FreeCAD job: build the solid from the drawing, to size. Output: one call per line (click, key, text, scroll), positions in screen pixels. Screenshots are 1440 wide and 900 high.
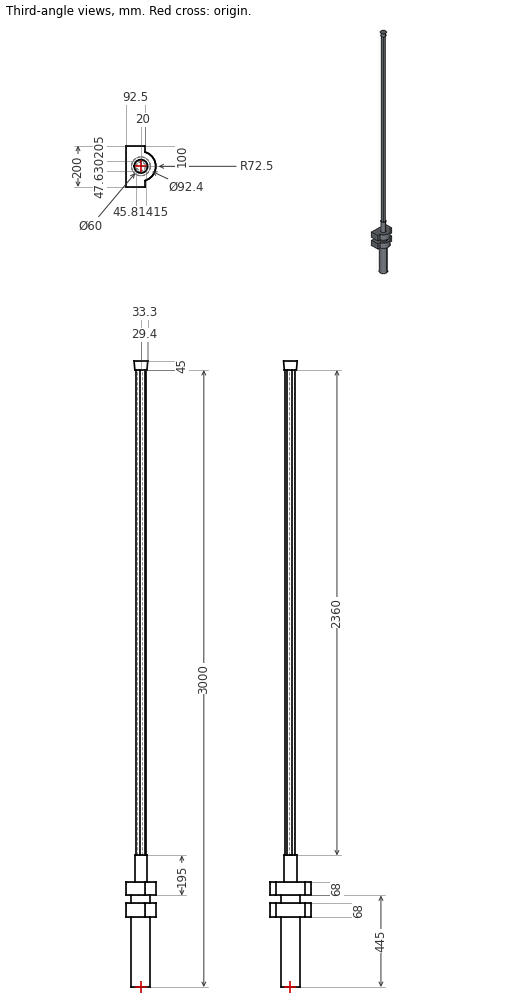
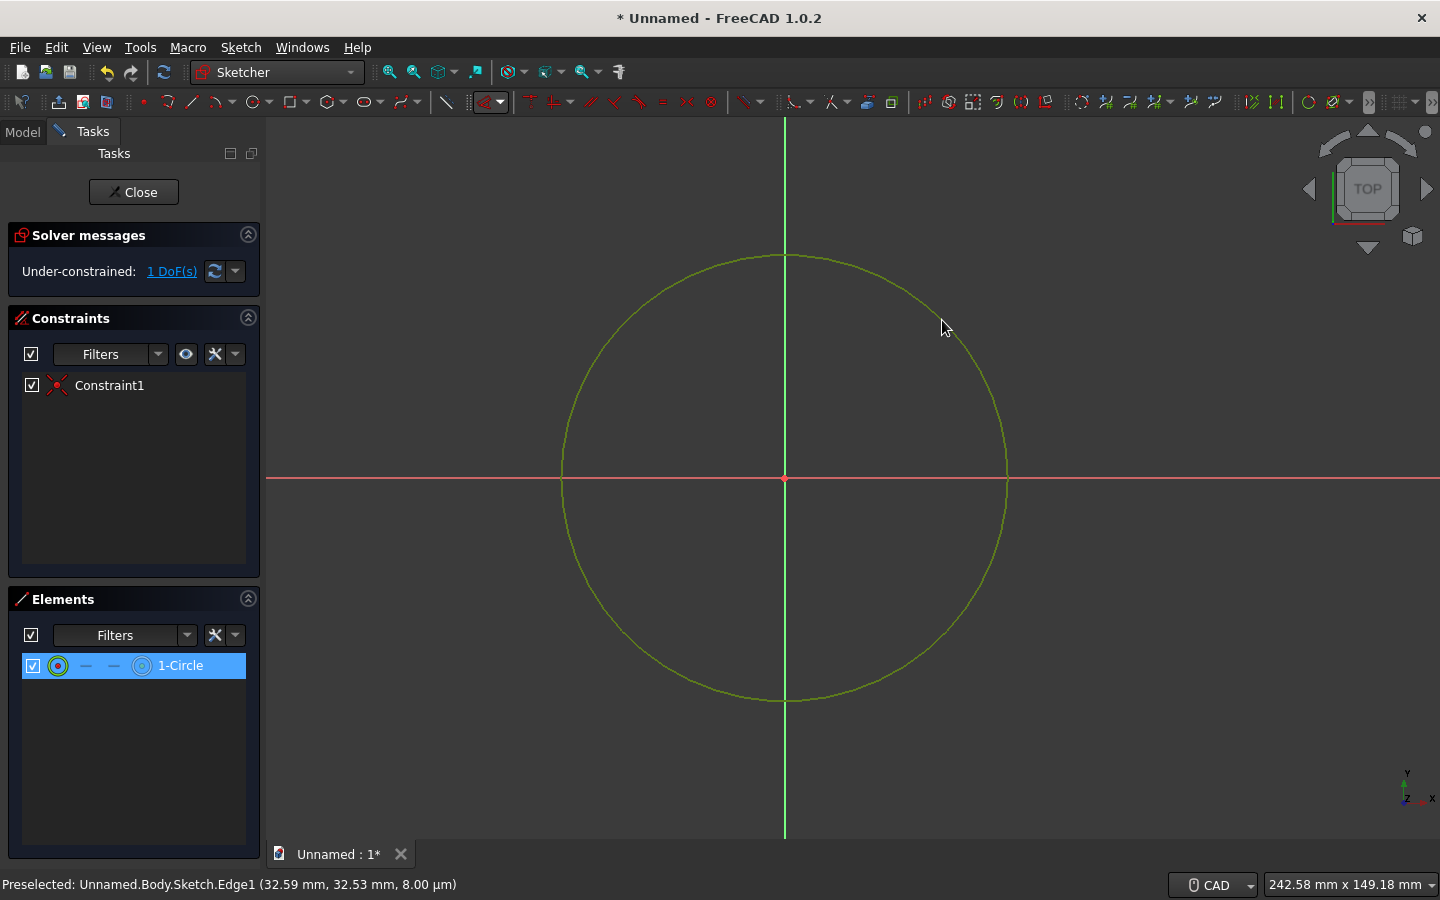
key(k)
key(o)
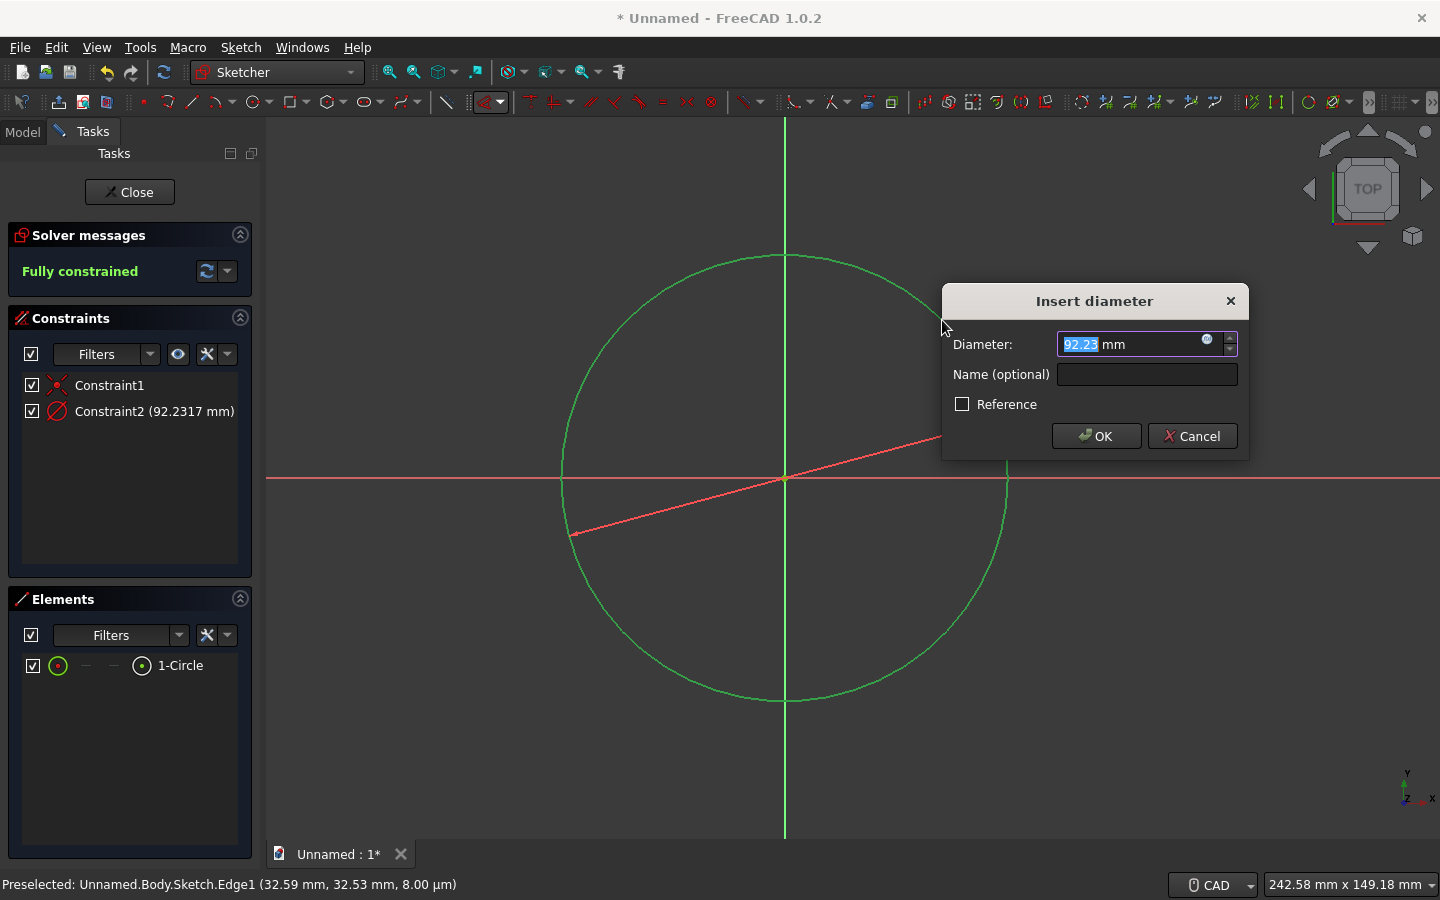
text(92.4)
key(Return)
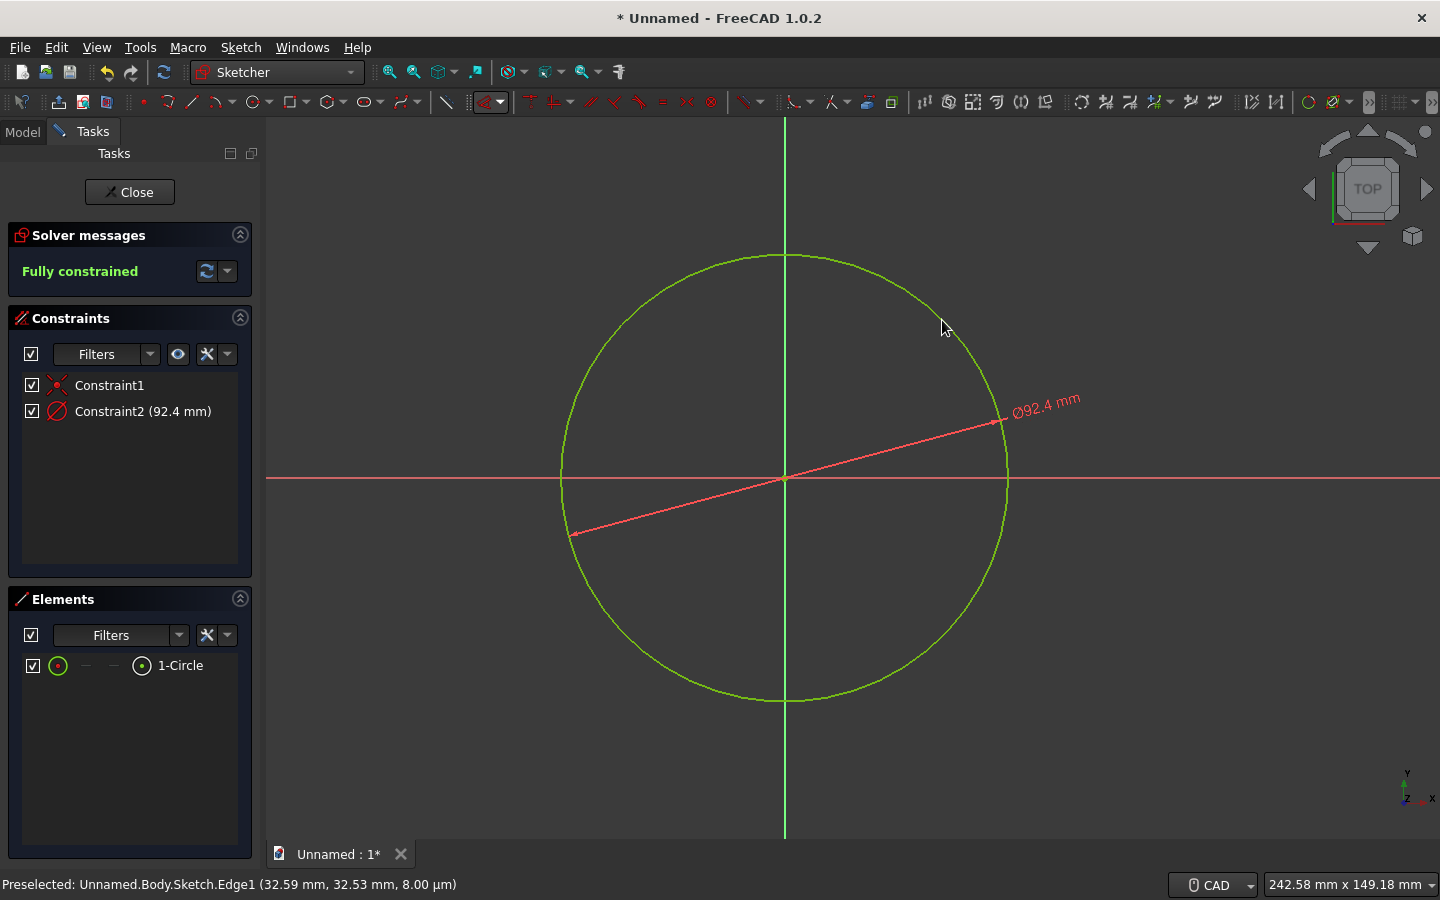
click(130, 192)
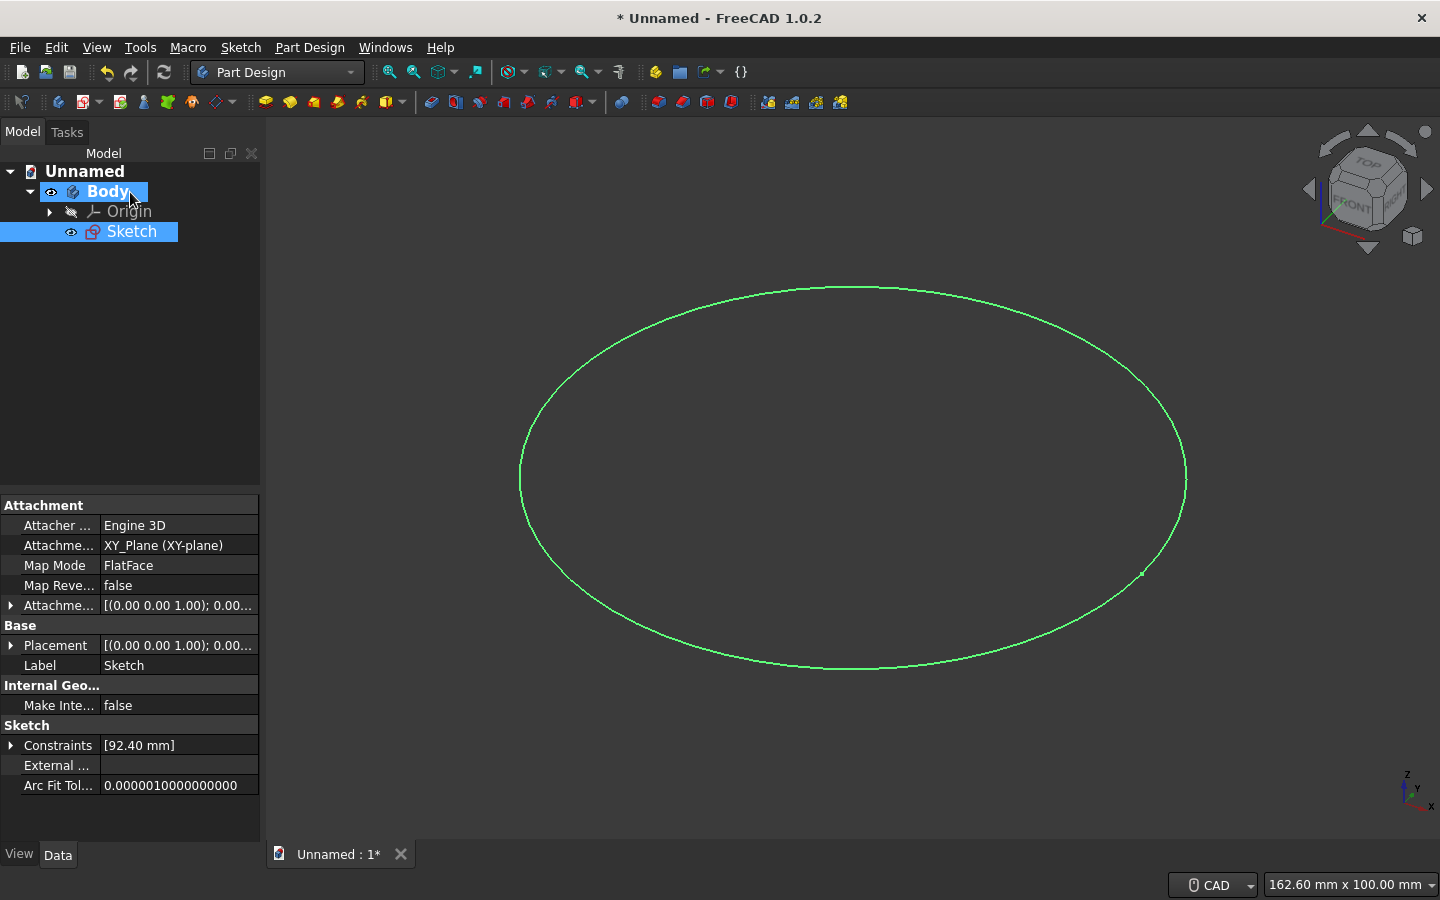
click(266, 102)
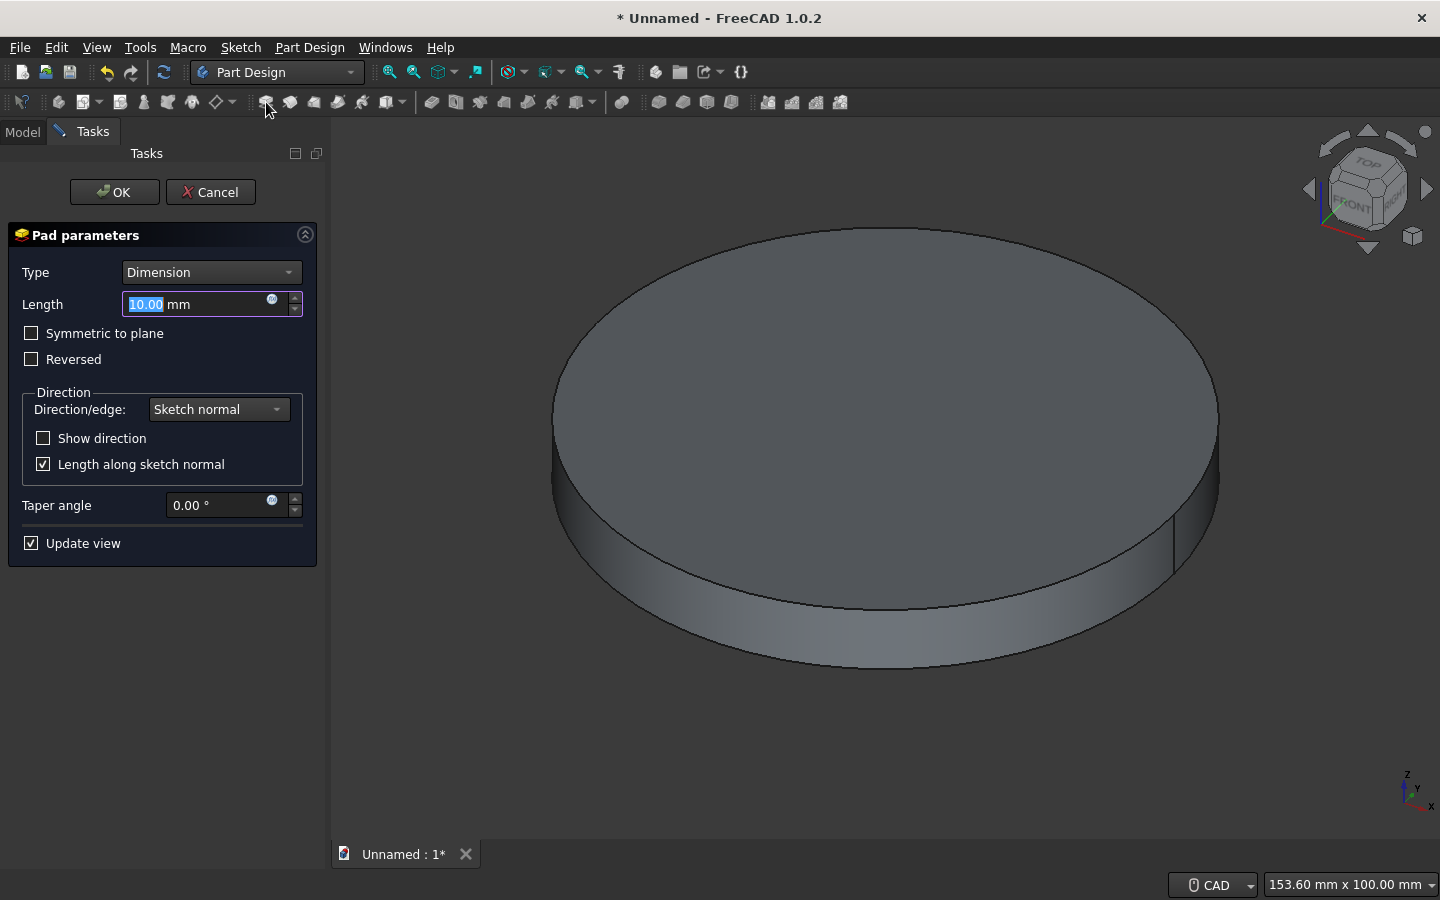
text(445)
key(Tab)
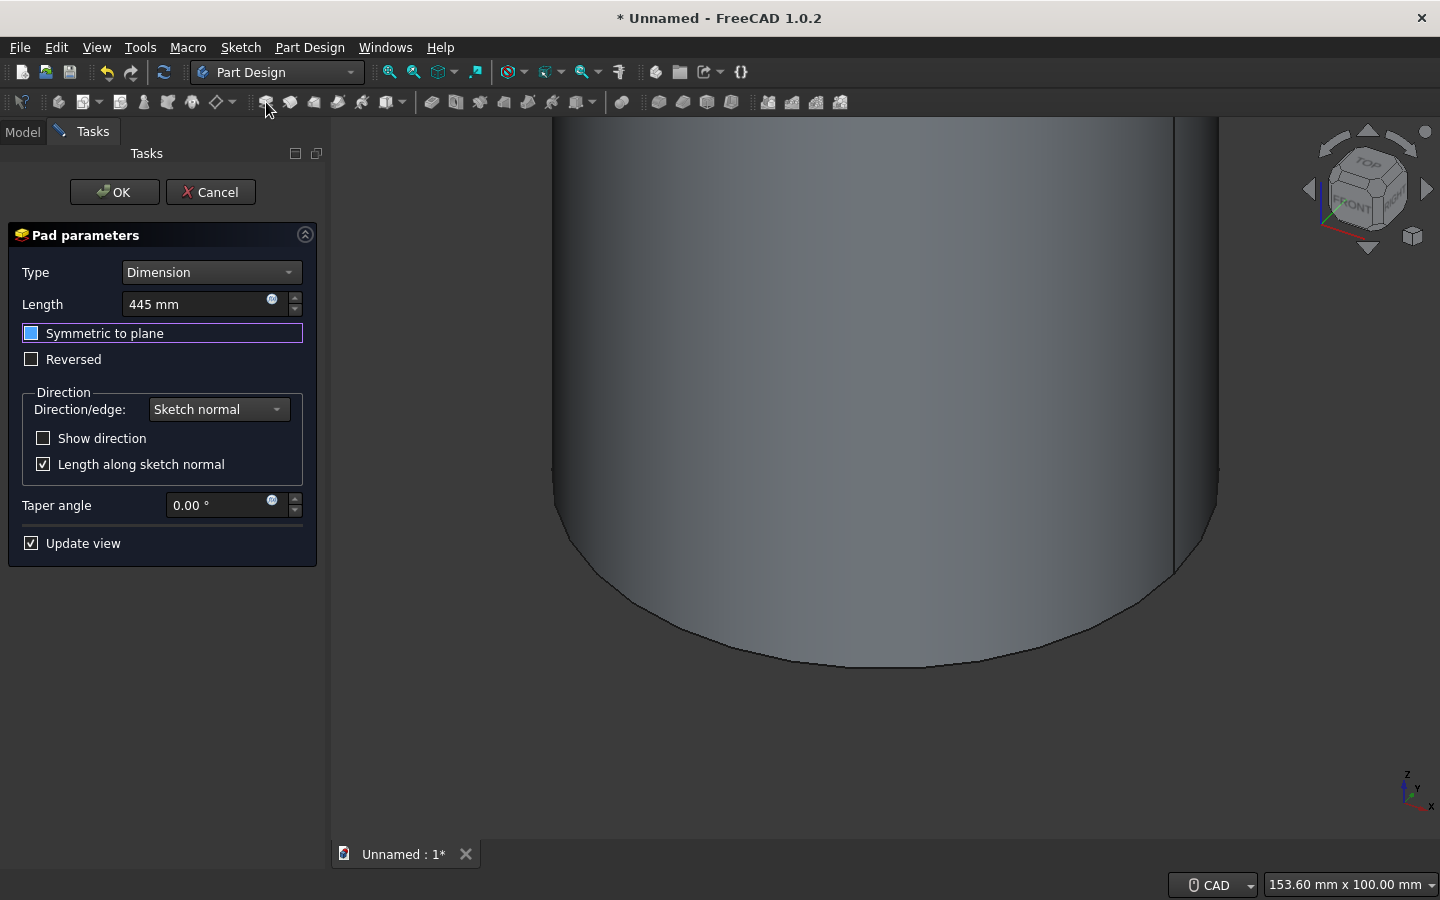
click(115, 192)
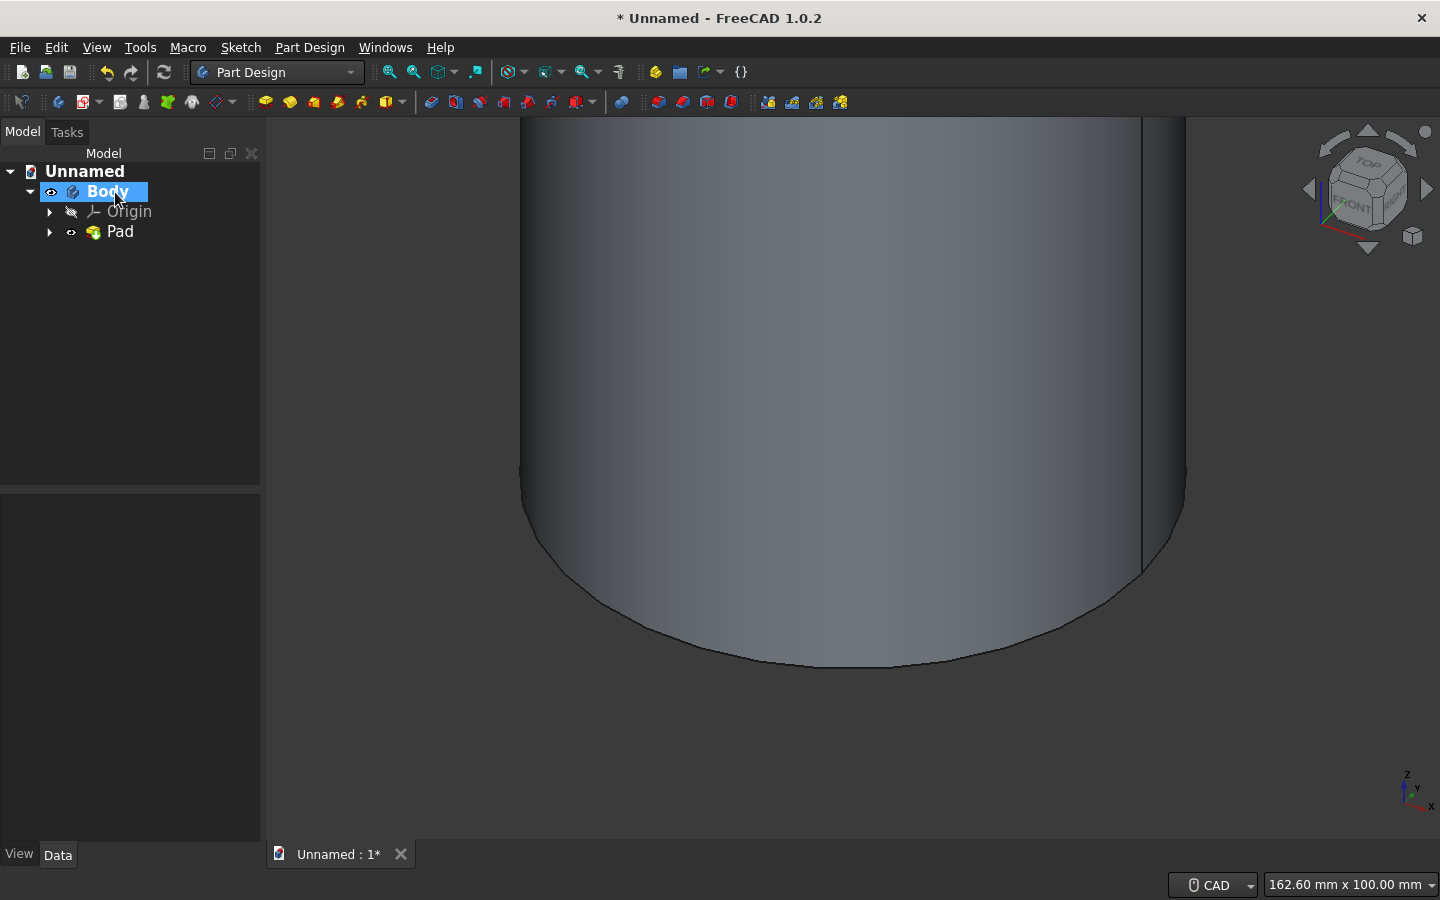
key(v)
key(f)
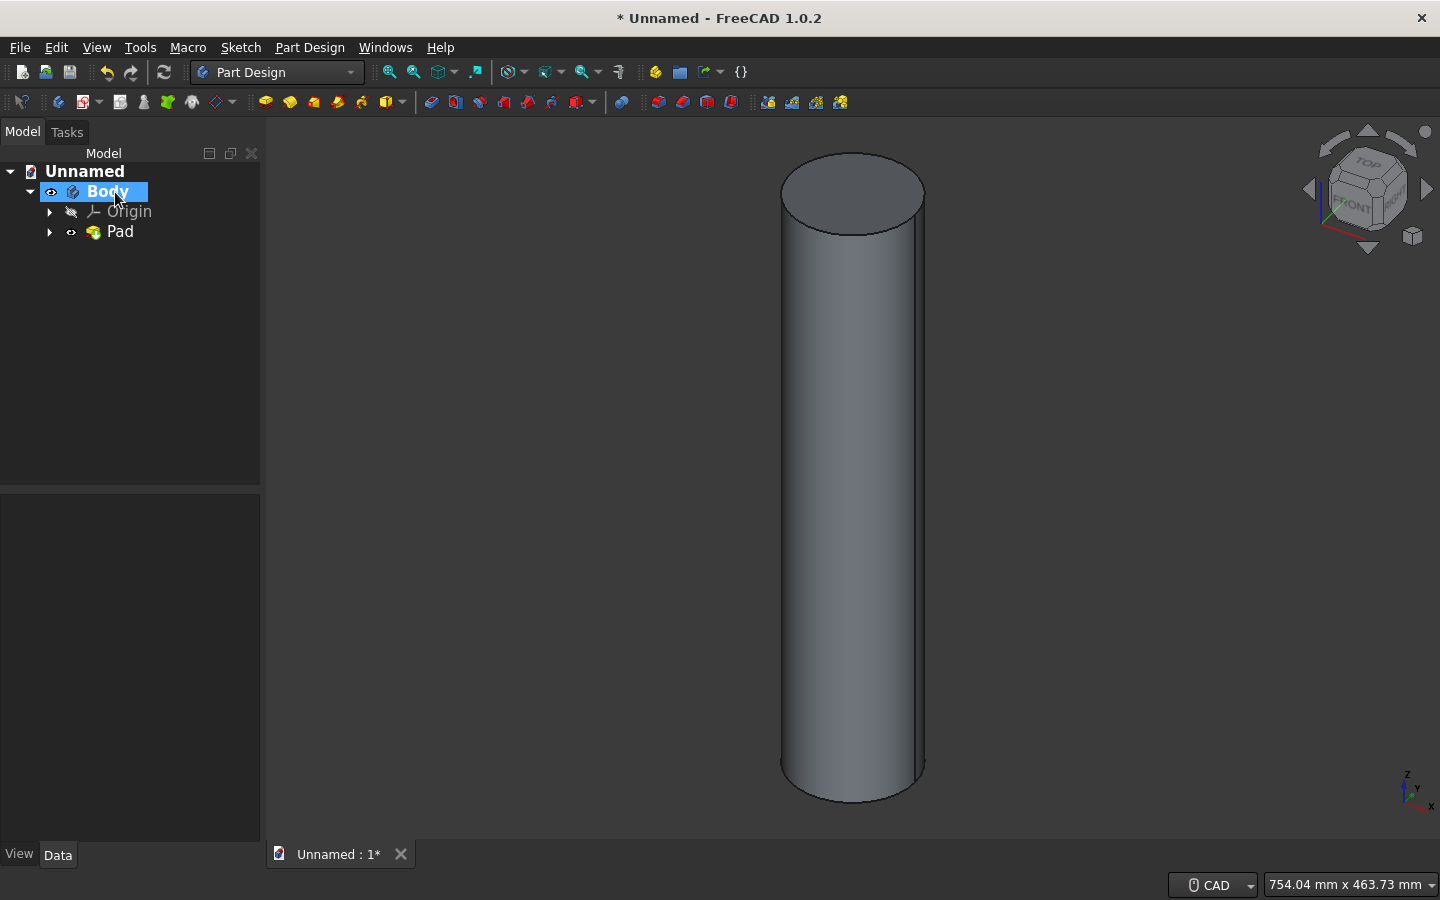
click(853, 193)